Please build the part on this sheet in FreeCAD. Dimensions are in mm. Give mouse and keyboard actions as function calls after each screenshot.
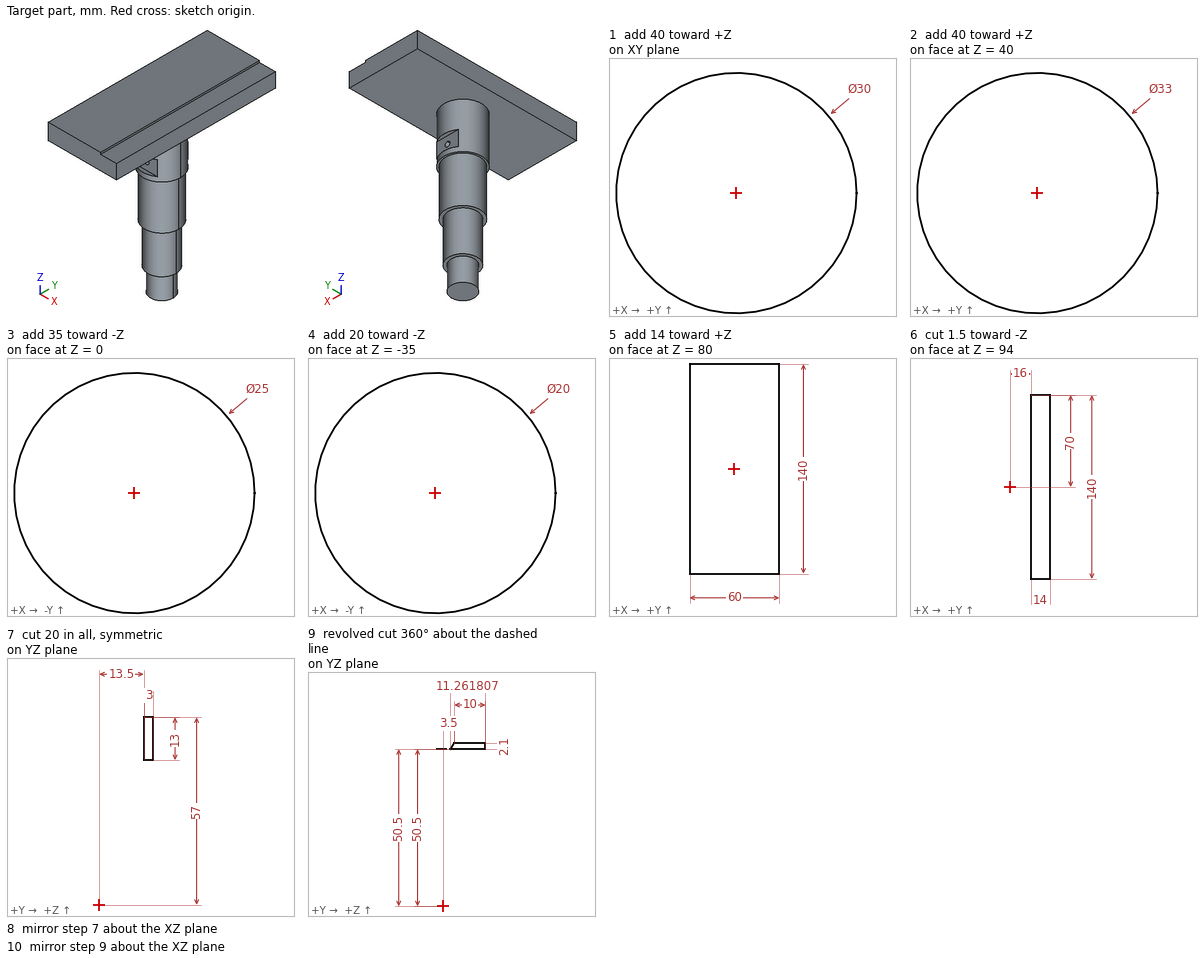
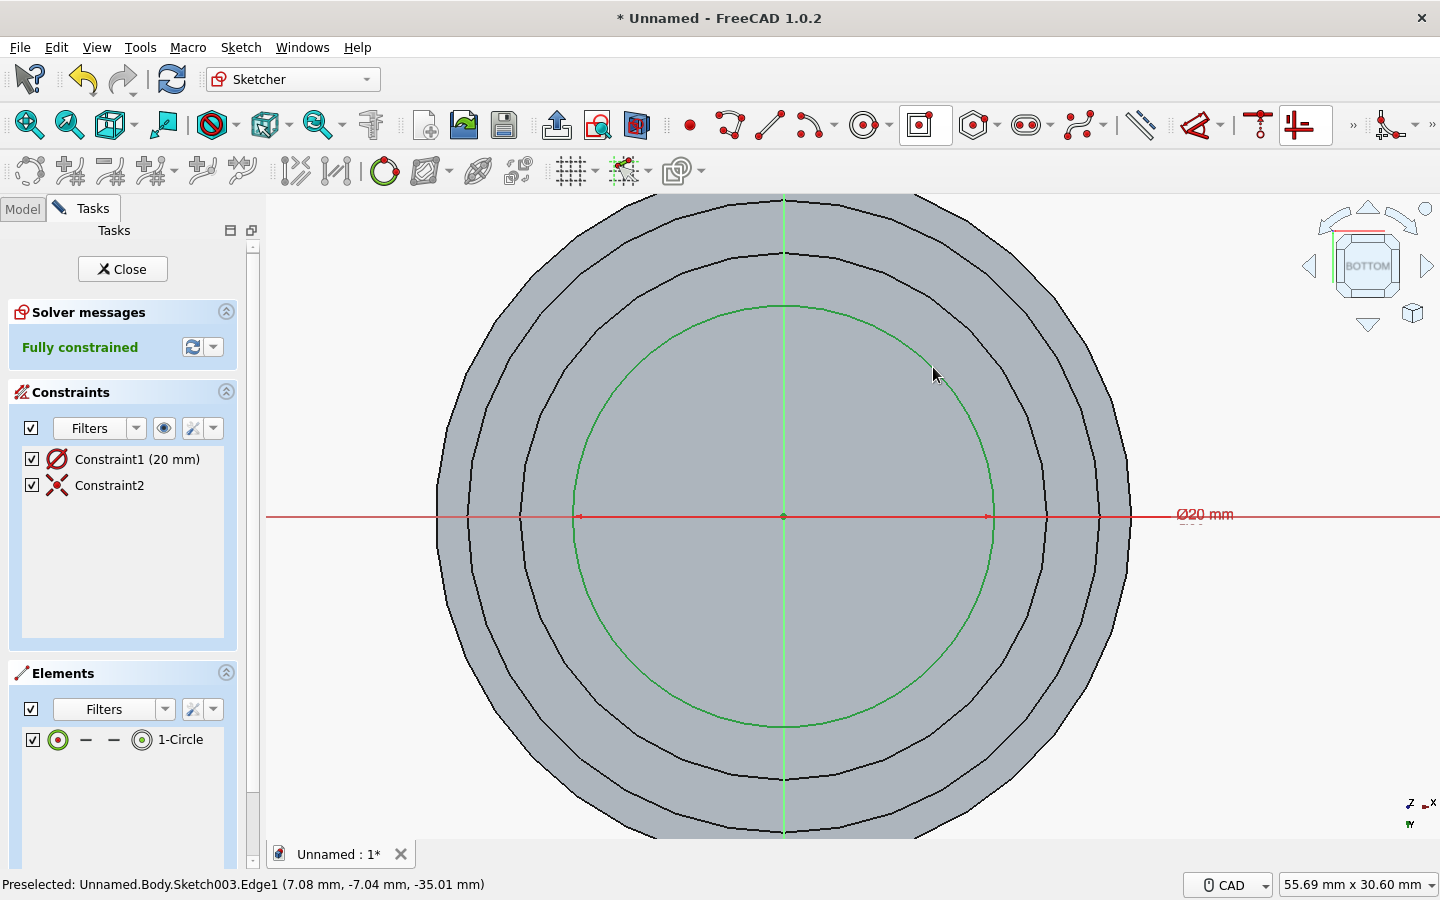
click(123, 269)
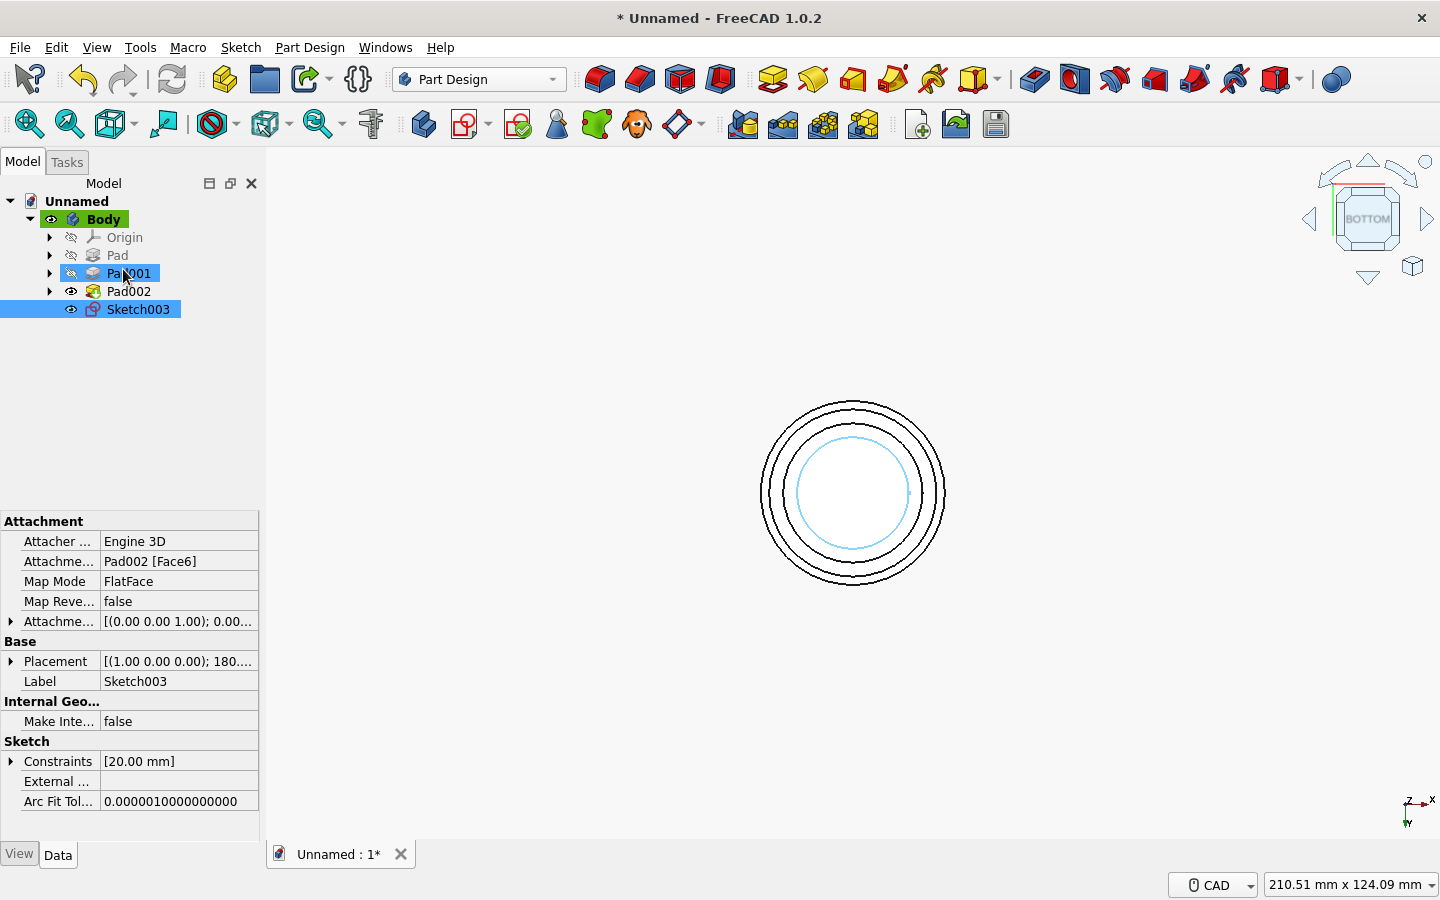
click(774, 80)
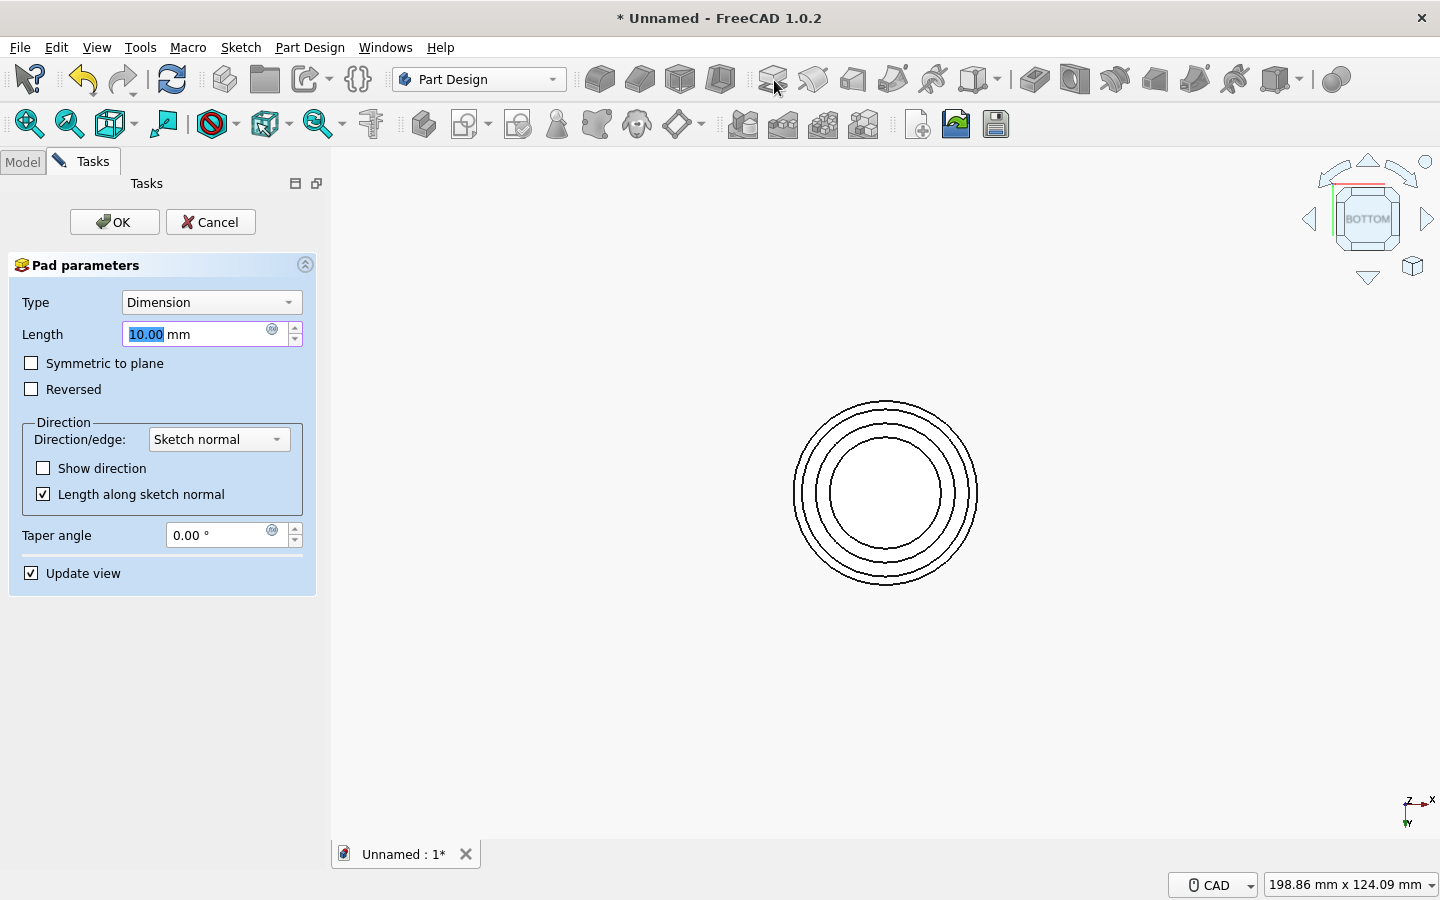
text(20)
key(Tab)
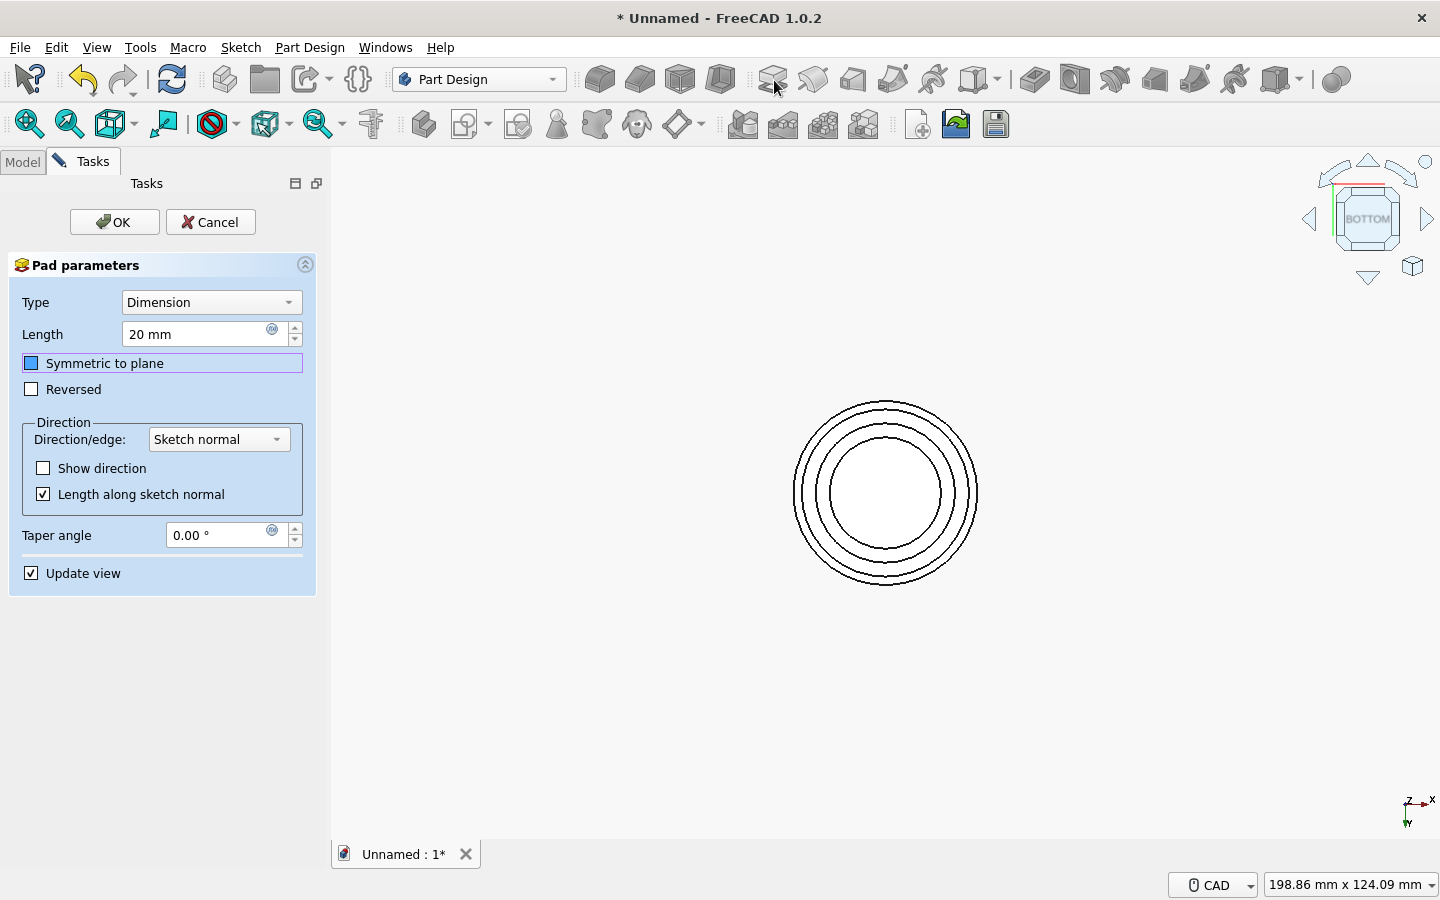
click(115, 222)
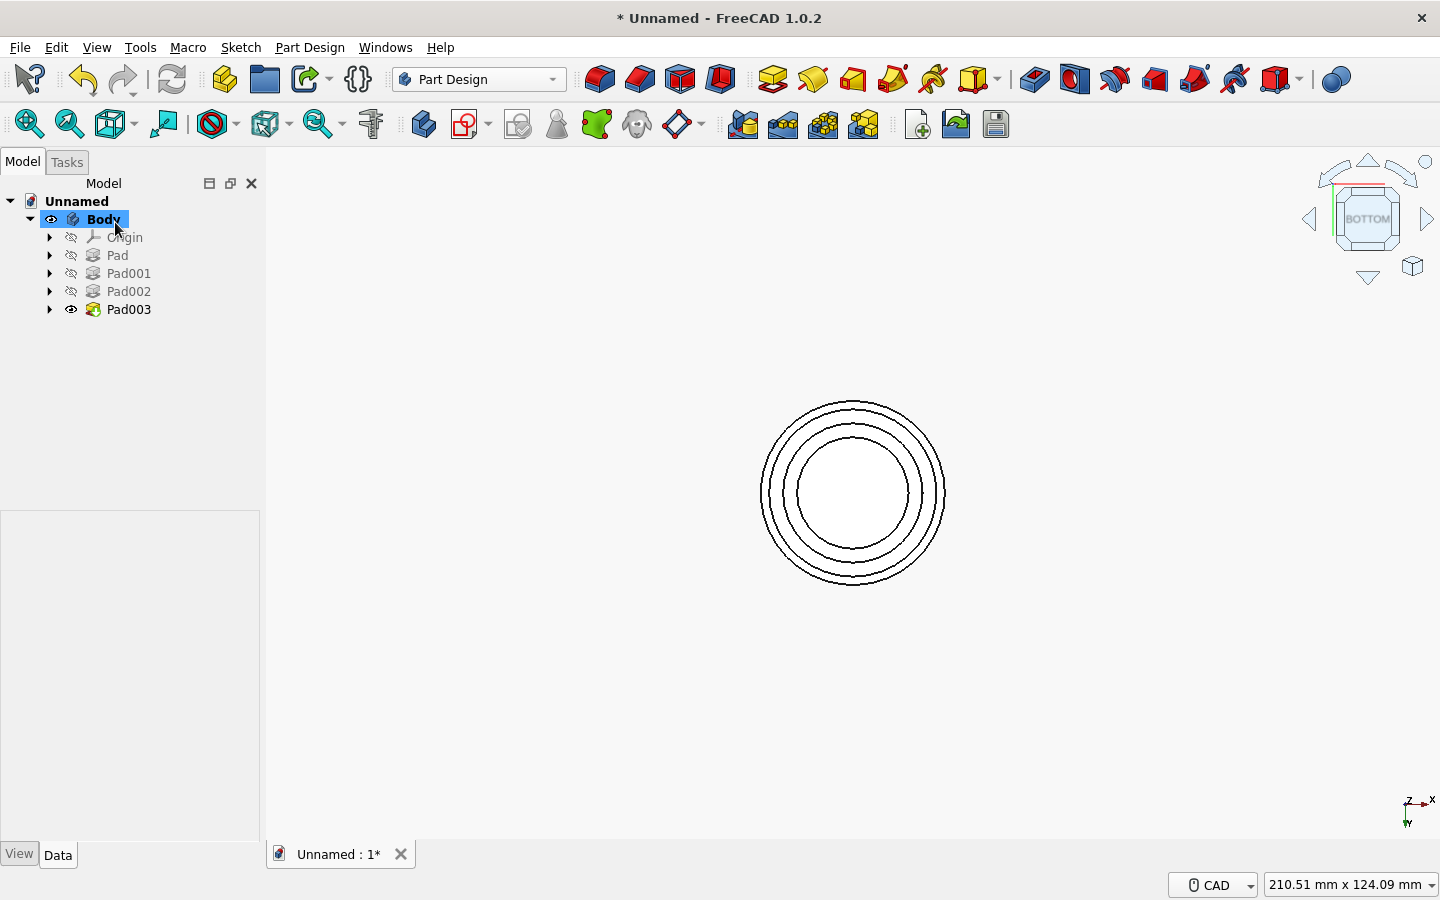
click(30, 124)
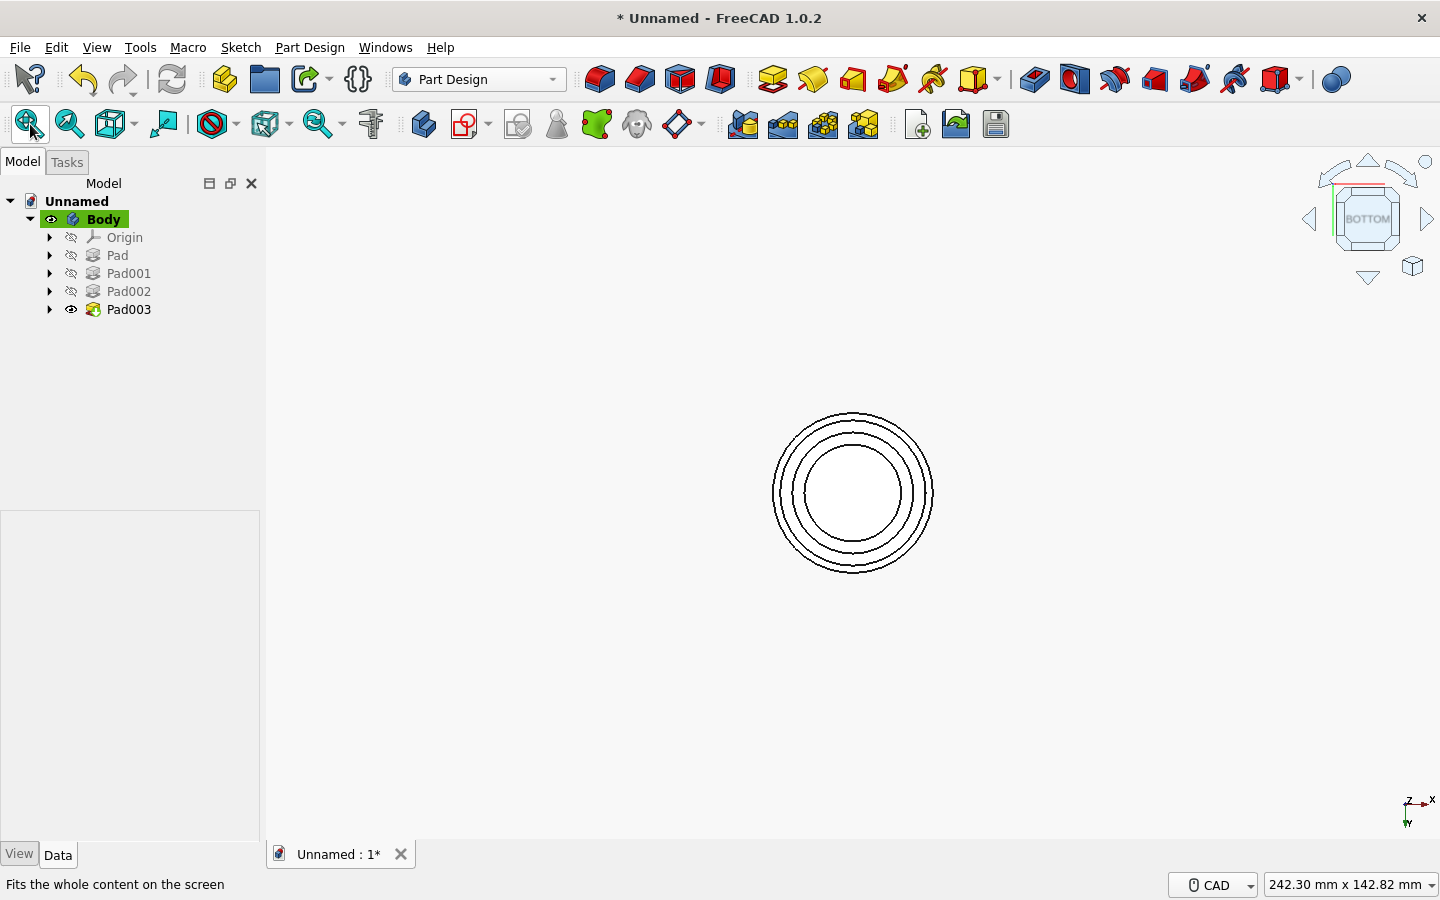
key(0)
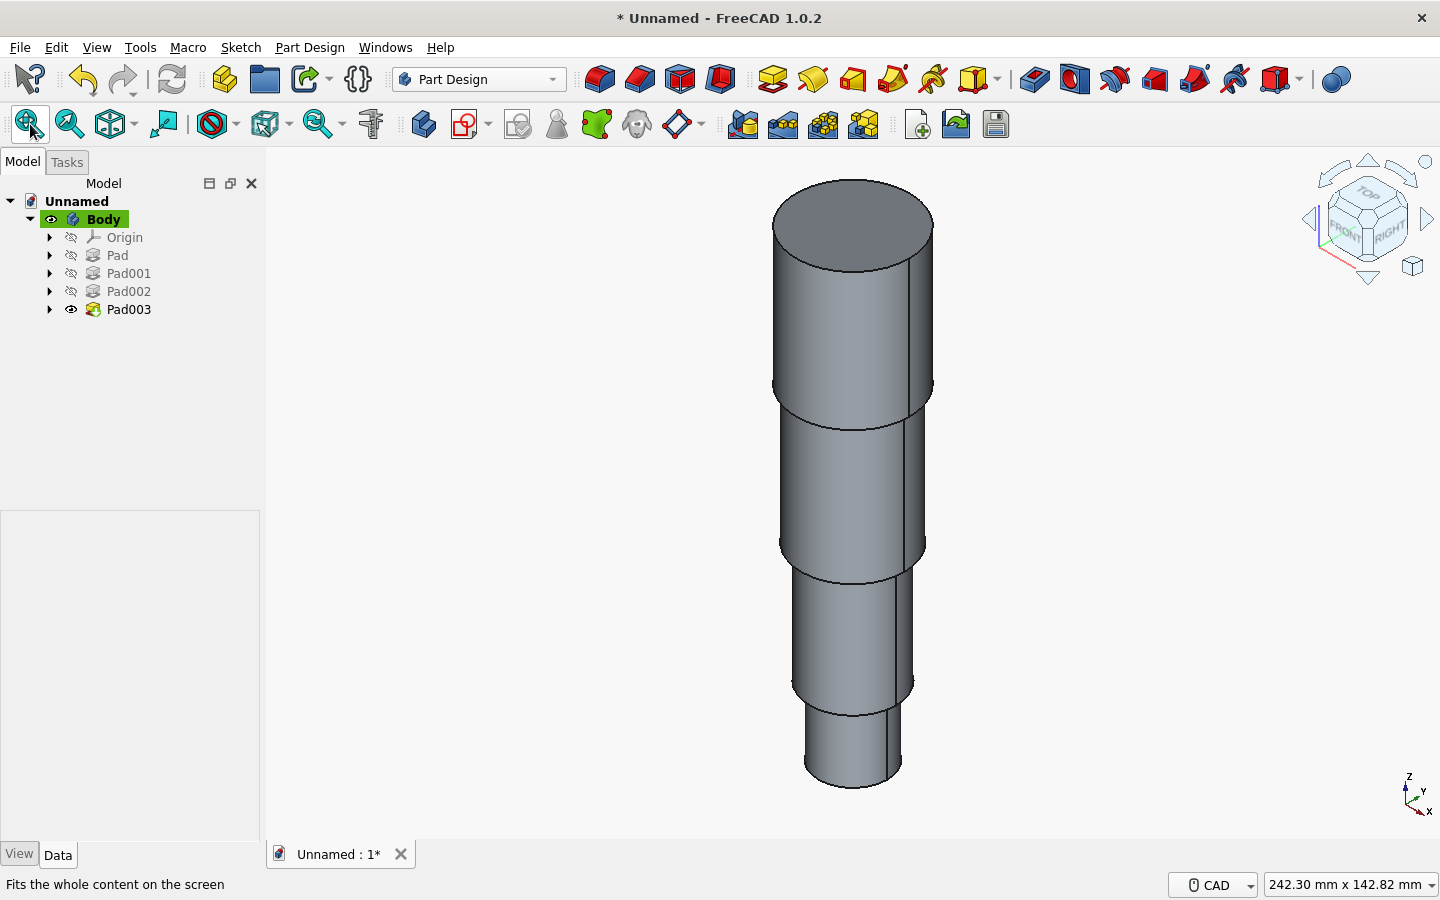
click(853, 225)